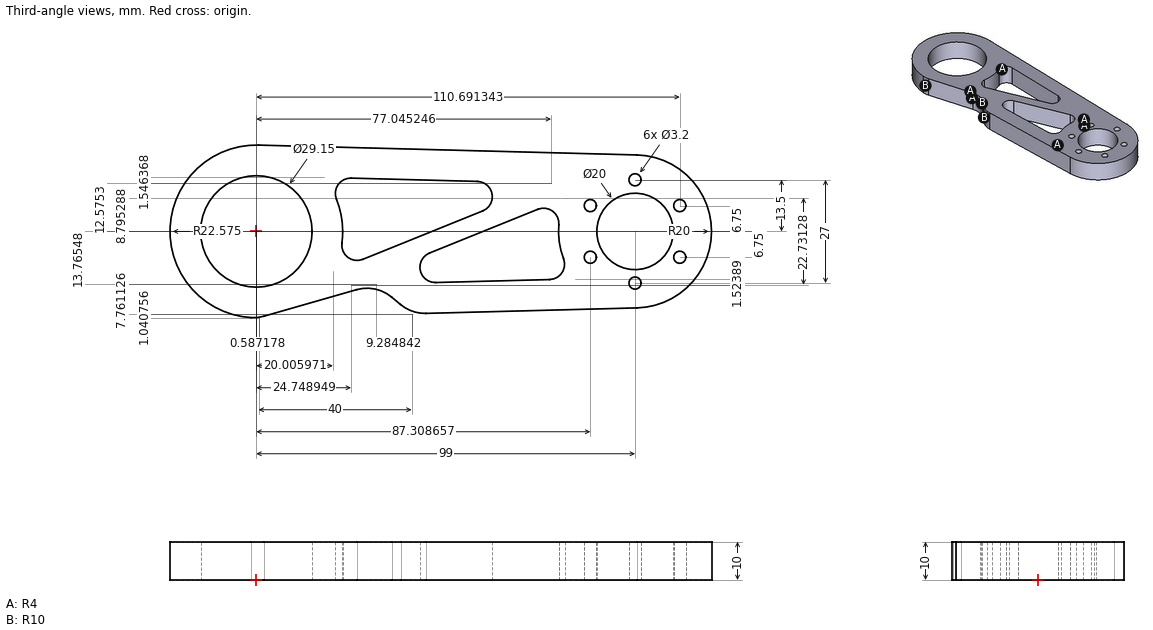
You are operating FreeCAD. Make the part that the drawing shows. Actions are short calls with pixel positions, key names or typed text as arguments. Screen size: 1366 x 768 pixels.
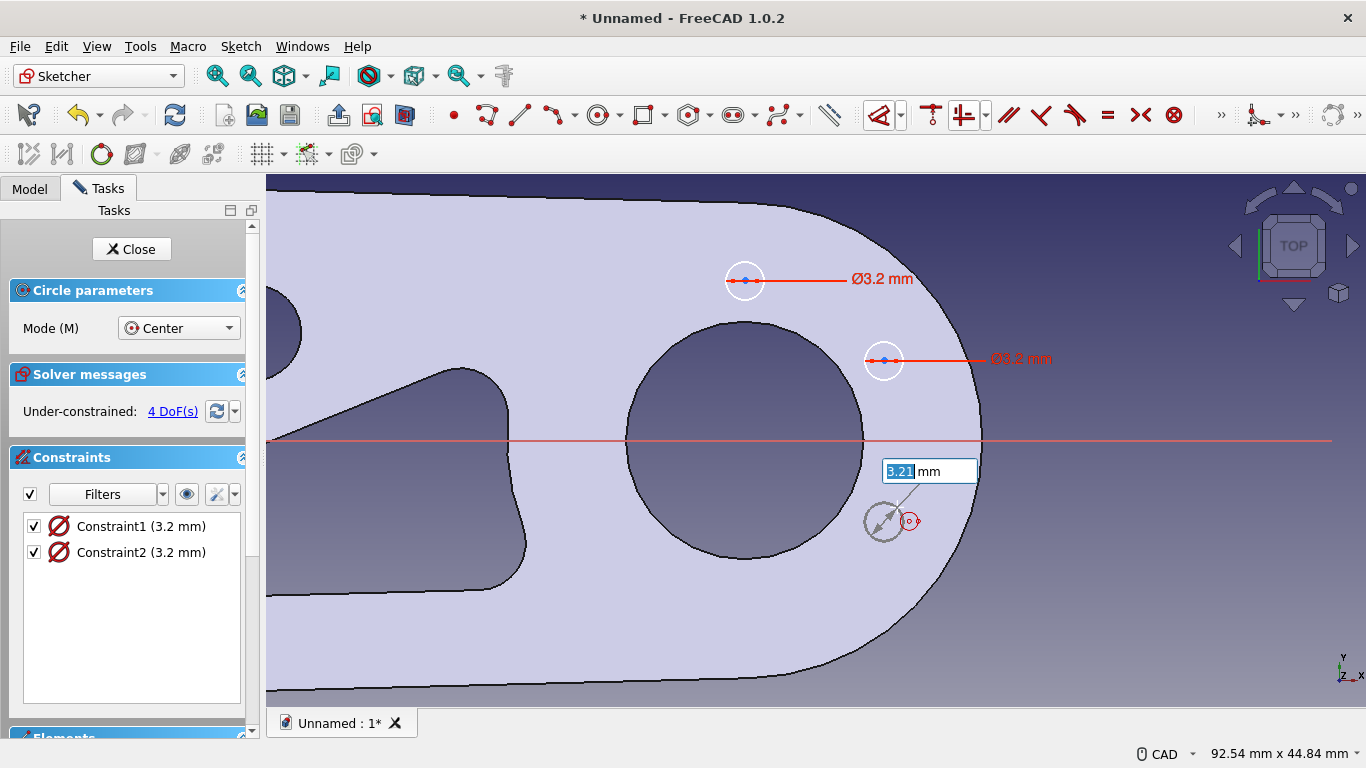
text(3.2)
key(Return)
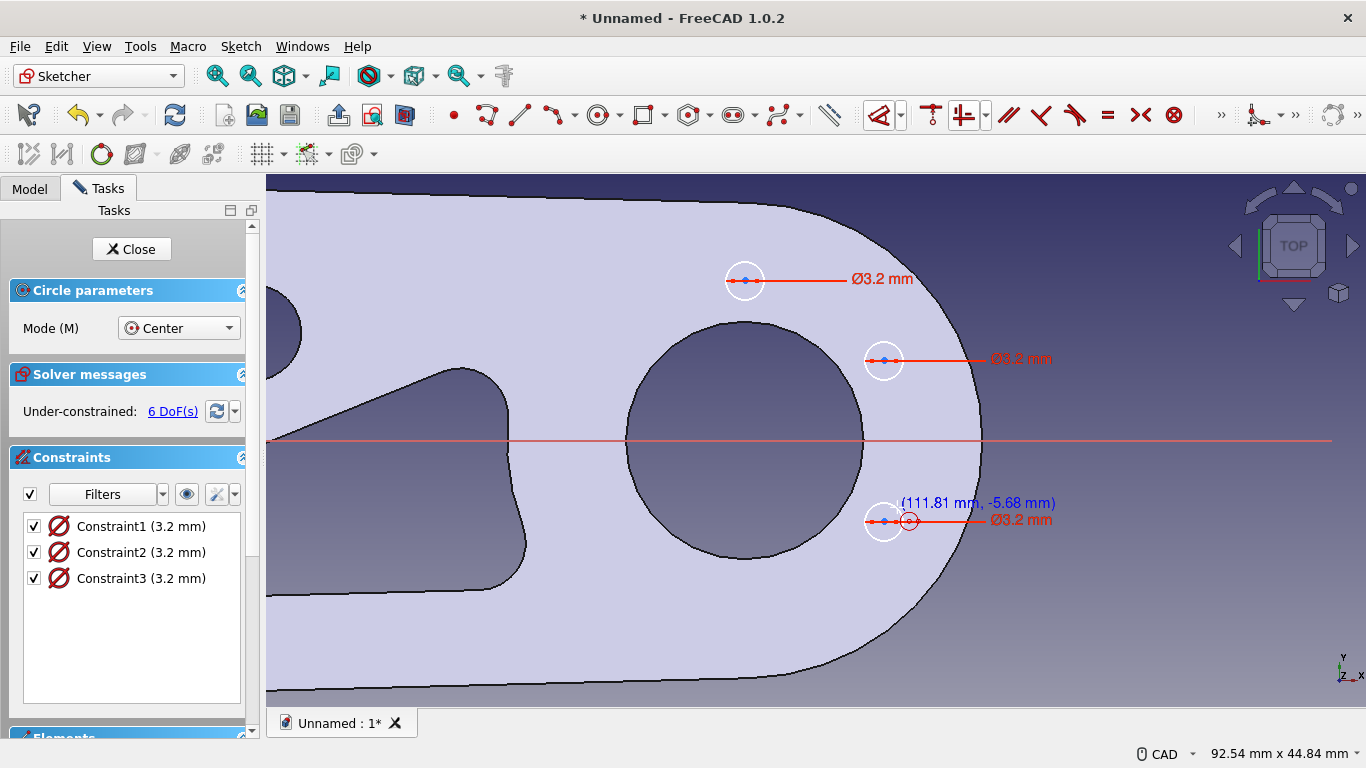
click(745, 601)
move(758, 588)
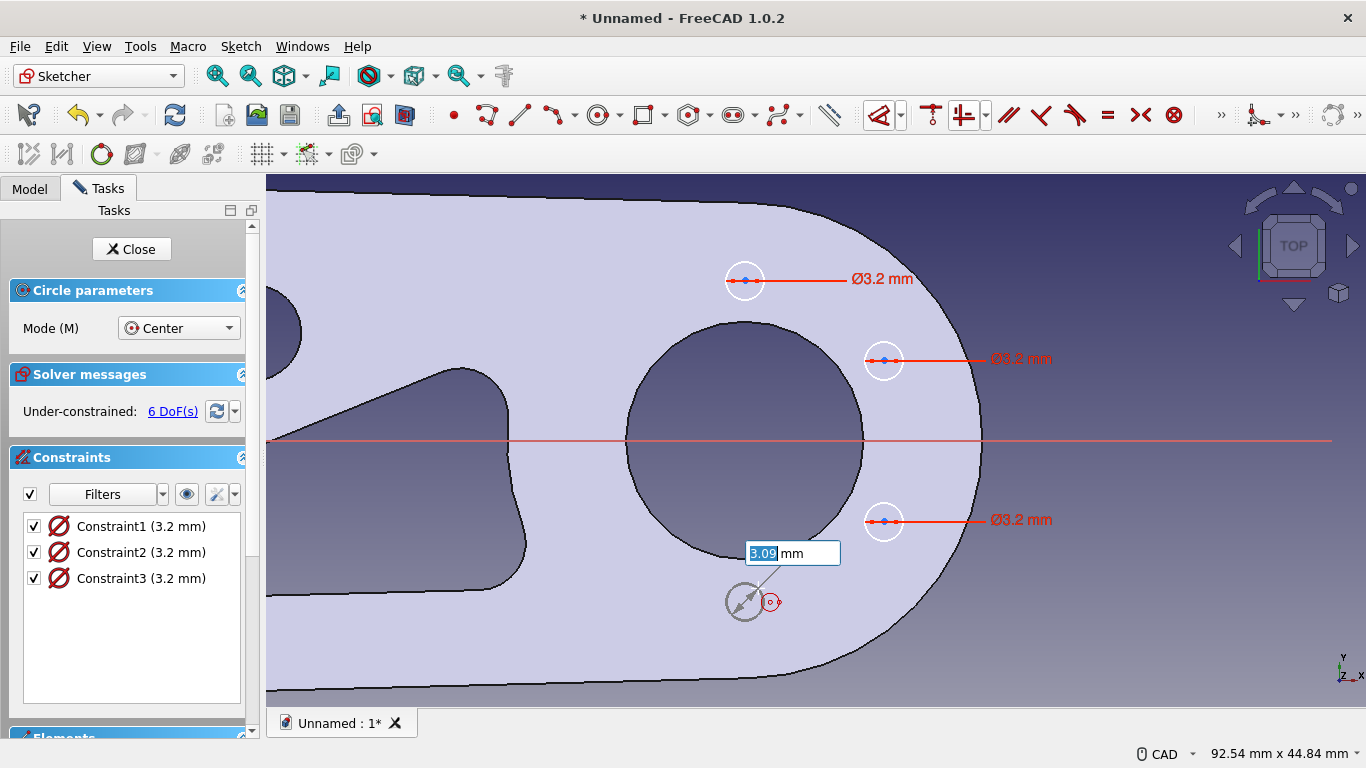
text(3.2)
key(Return)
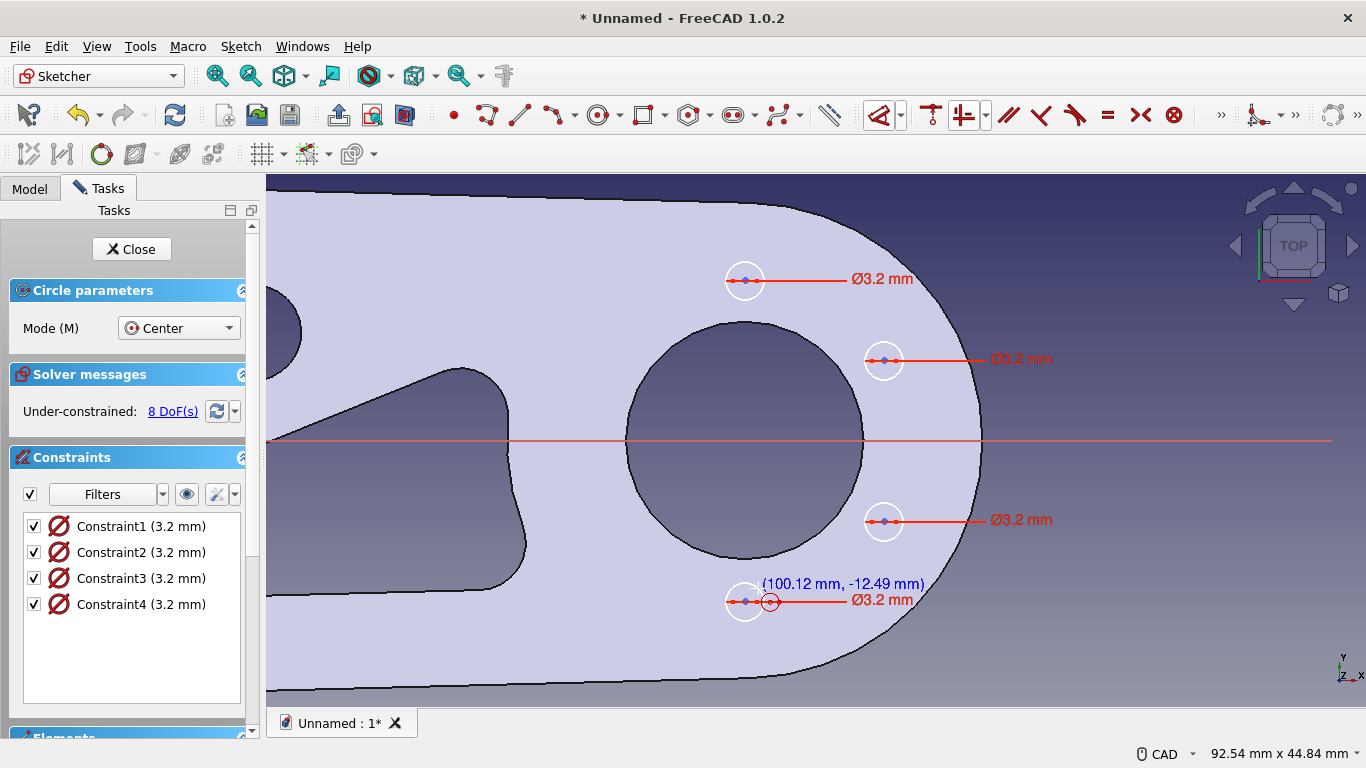
click(606, 521)
move(619, 507)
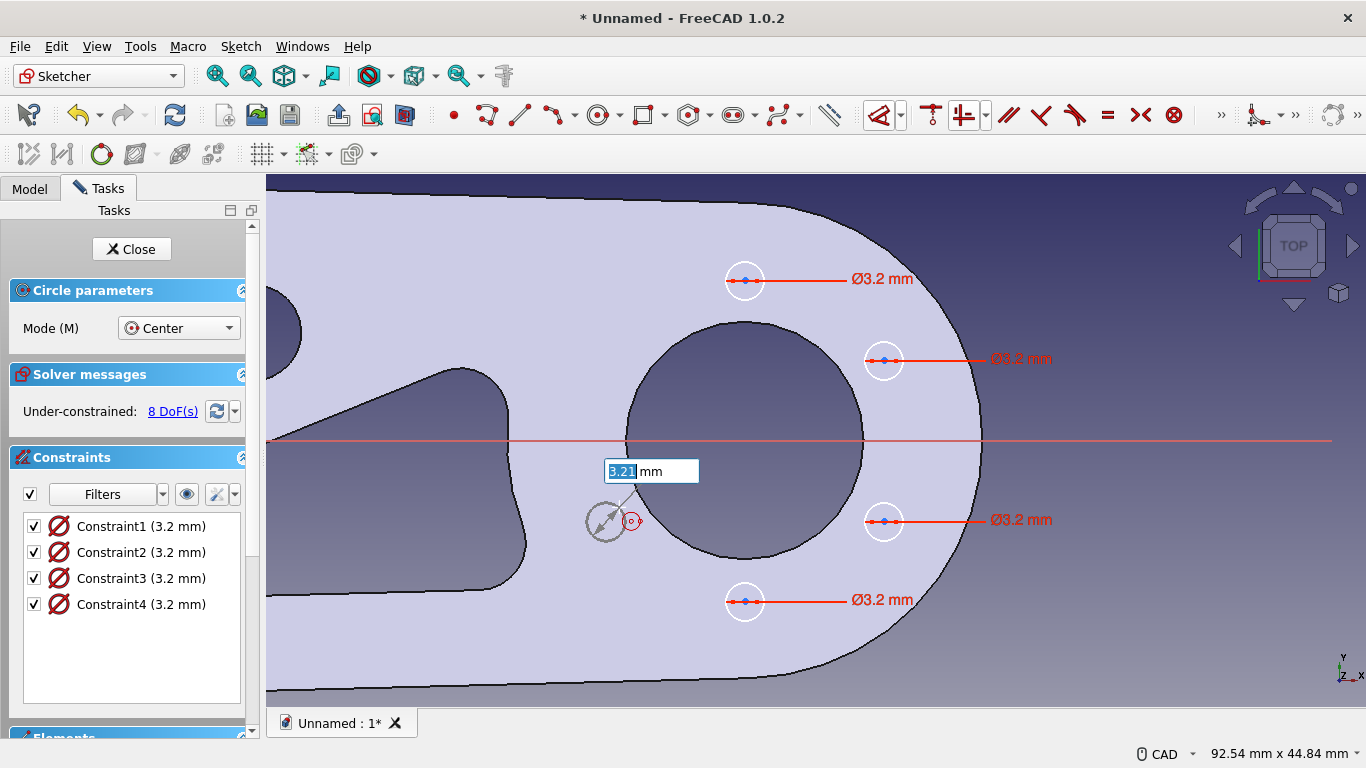
text(3.2)
key(Return)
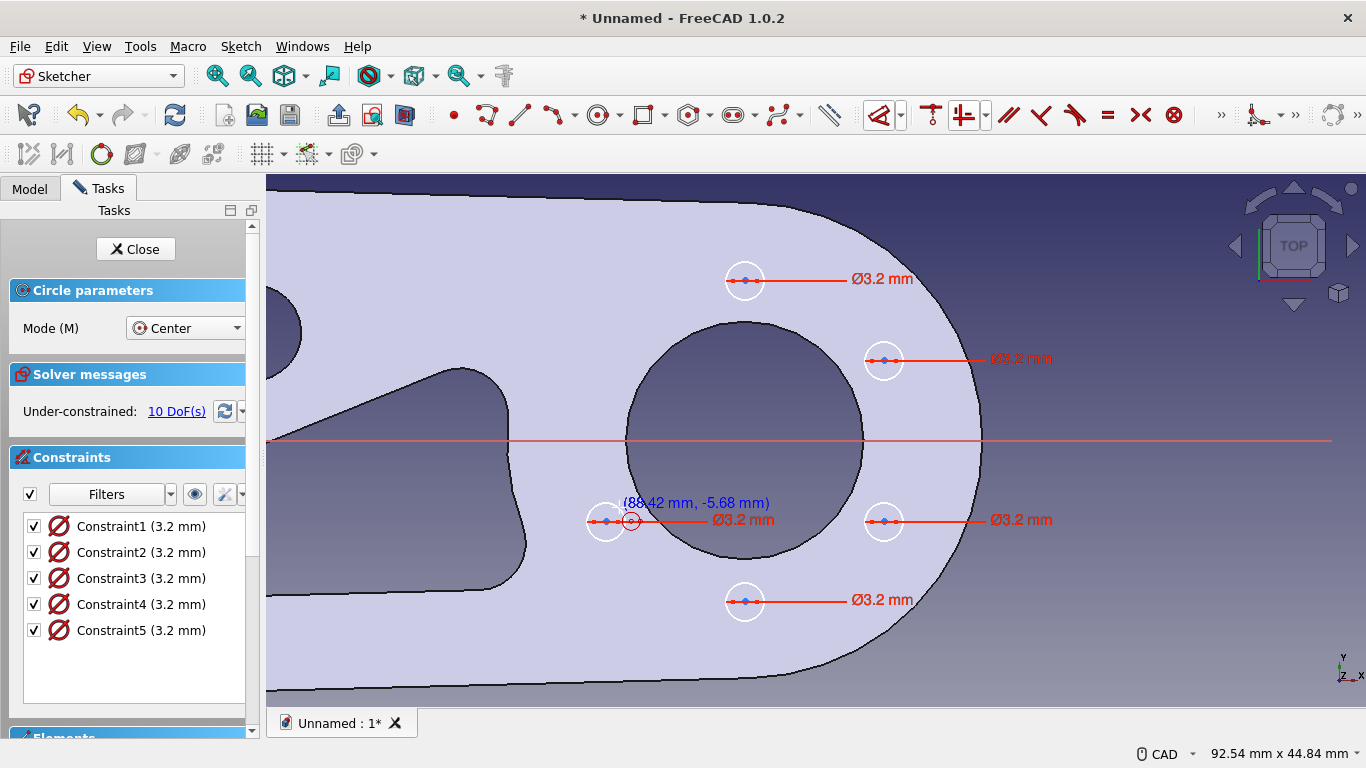
click(606, 360)
move(619, 347)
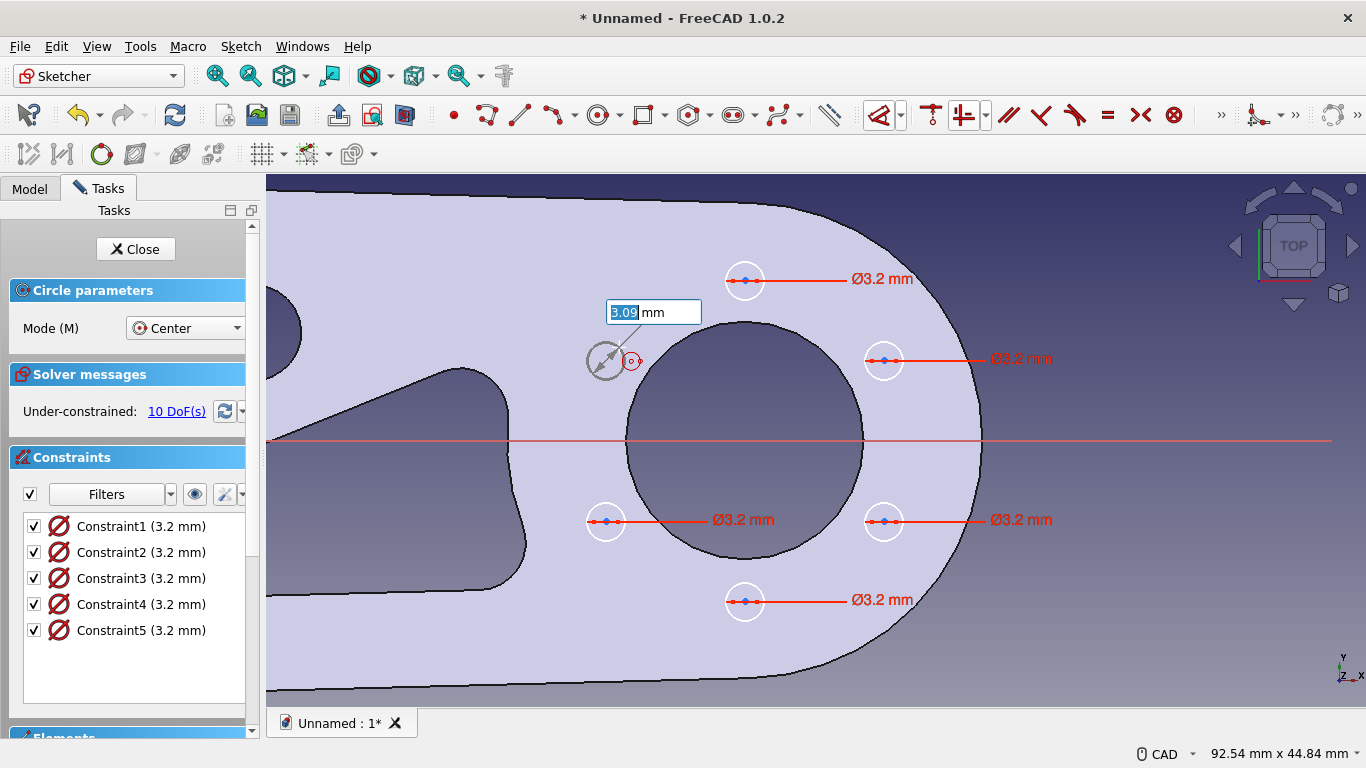
text(3.2)
key(Return)
key(Escape)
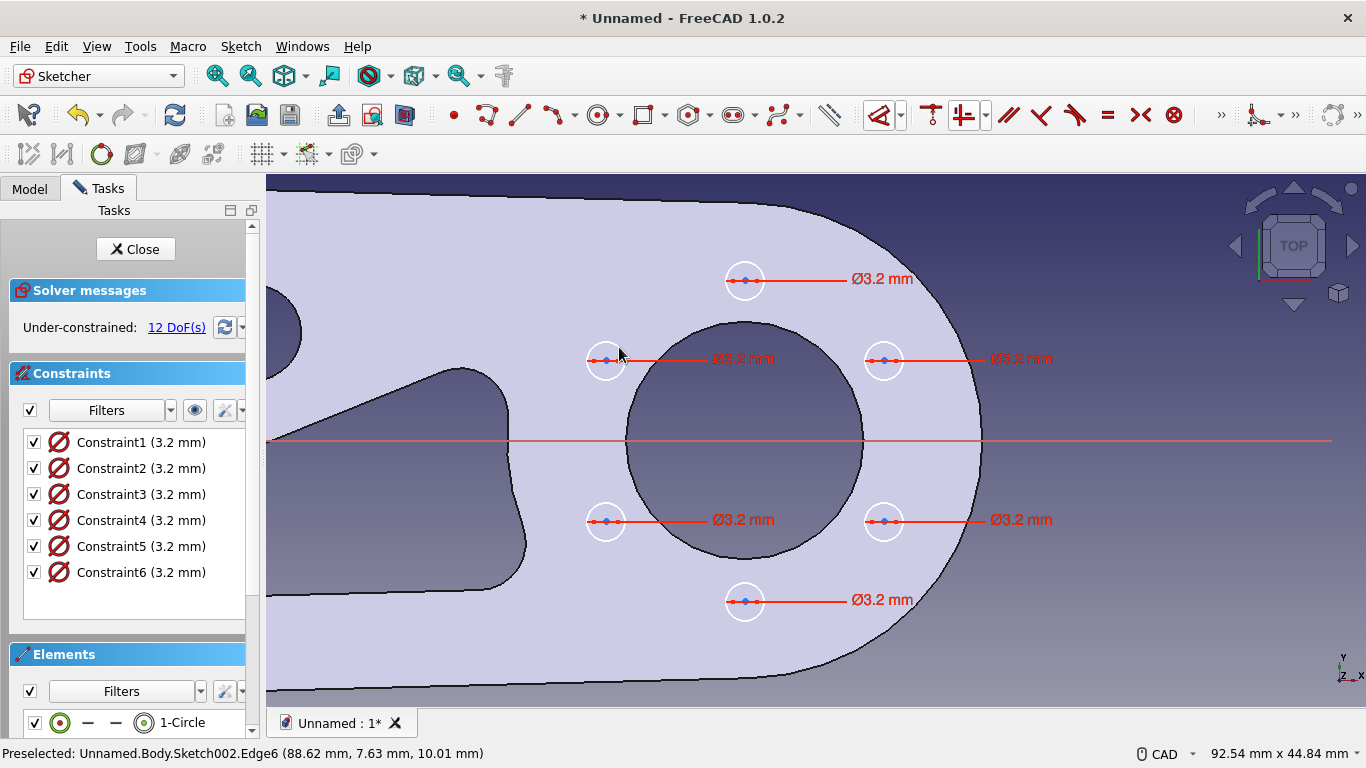
click(884, 361)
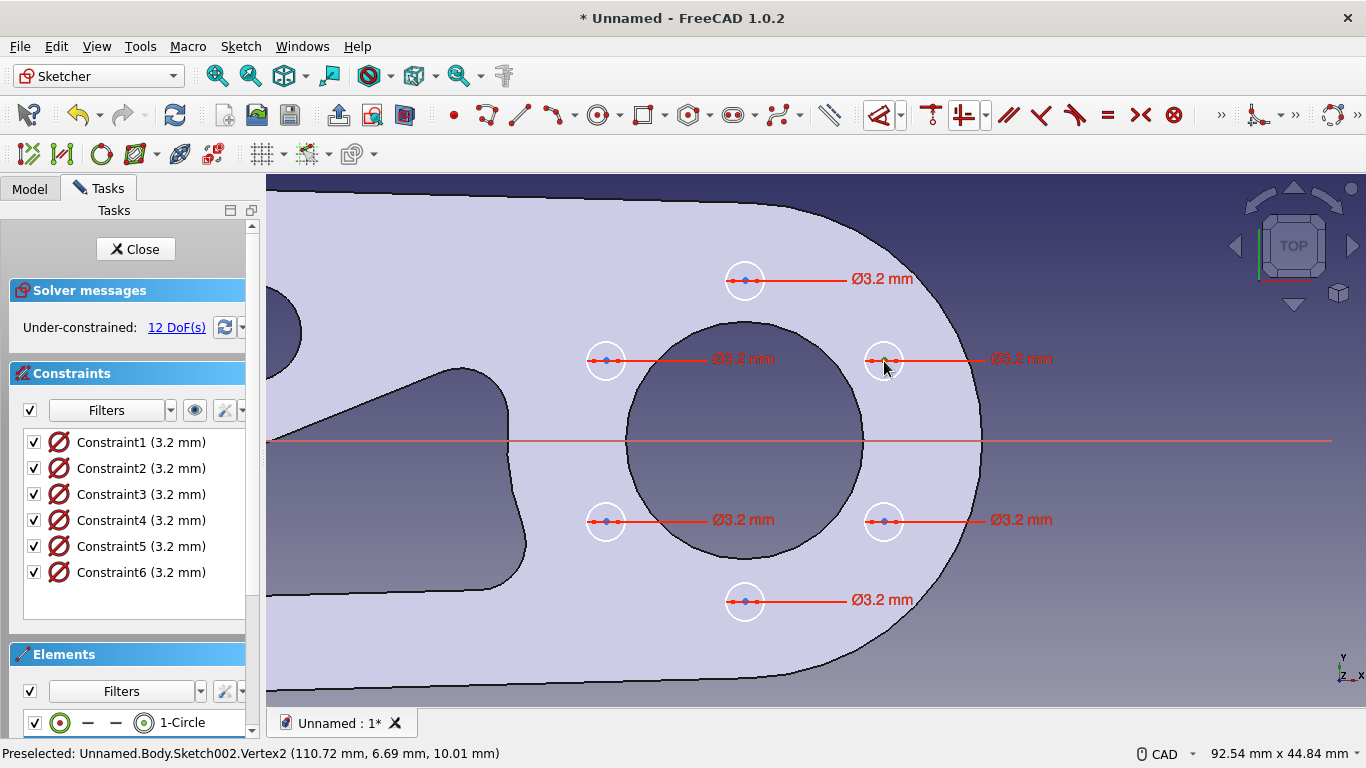
click(884, 522)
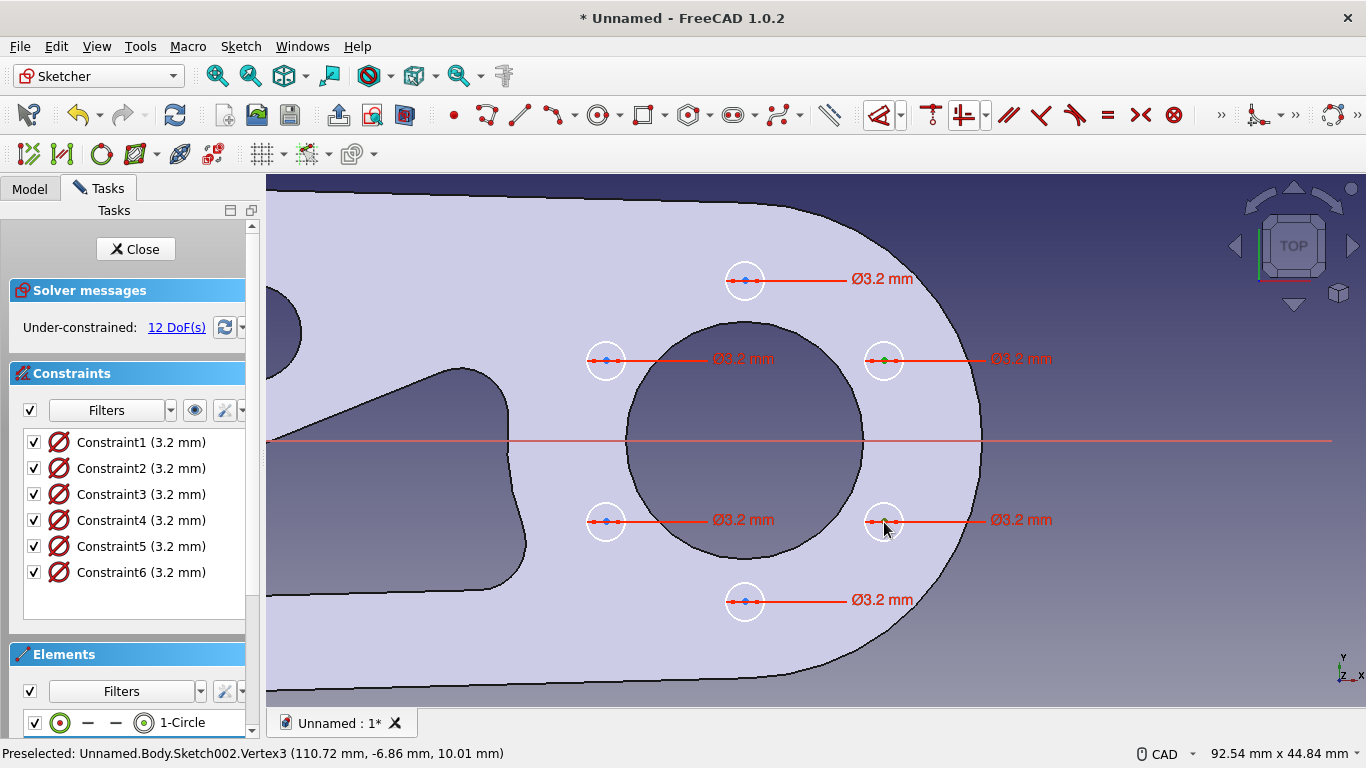
key(v)